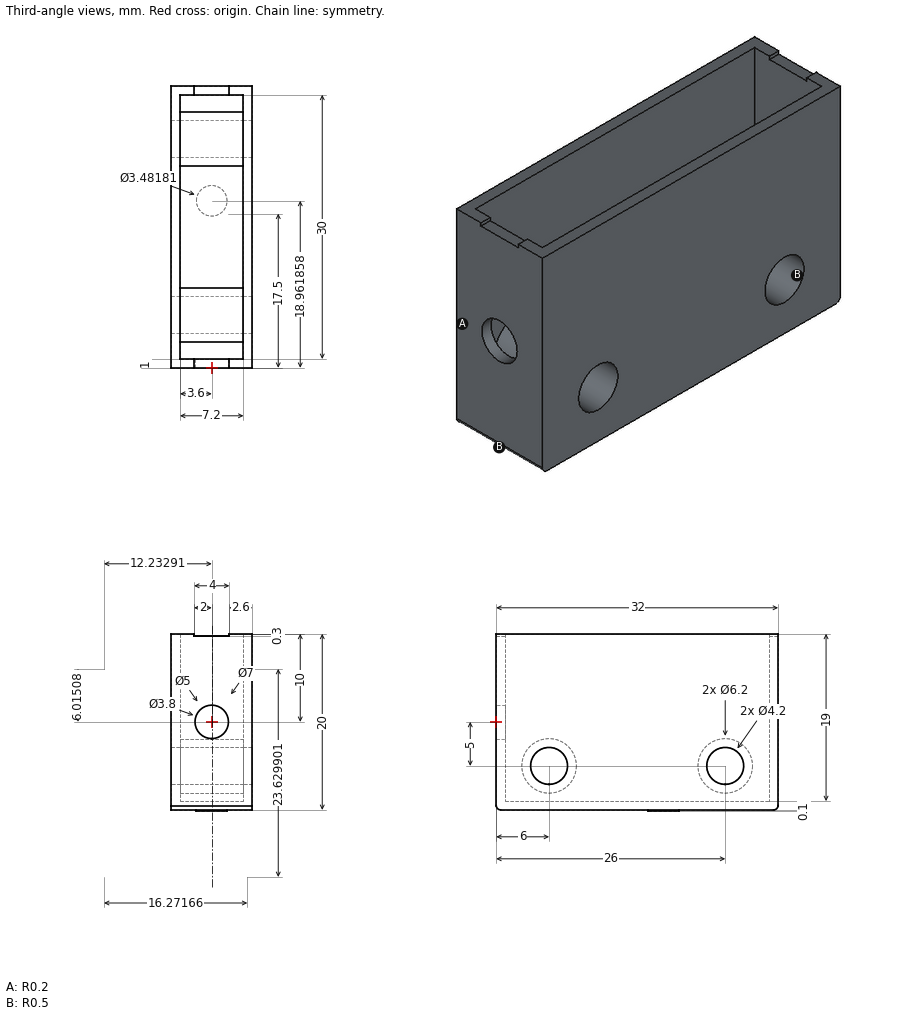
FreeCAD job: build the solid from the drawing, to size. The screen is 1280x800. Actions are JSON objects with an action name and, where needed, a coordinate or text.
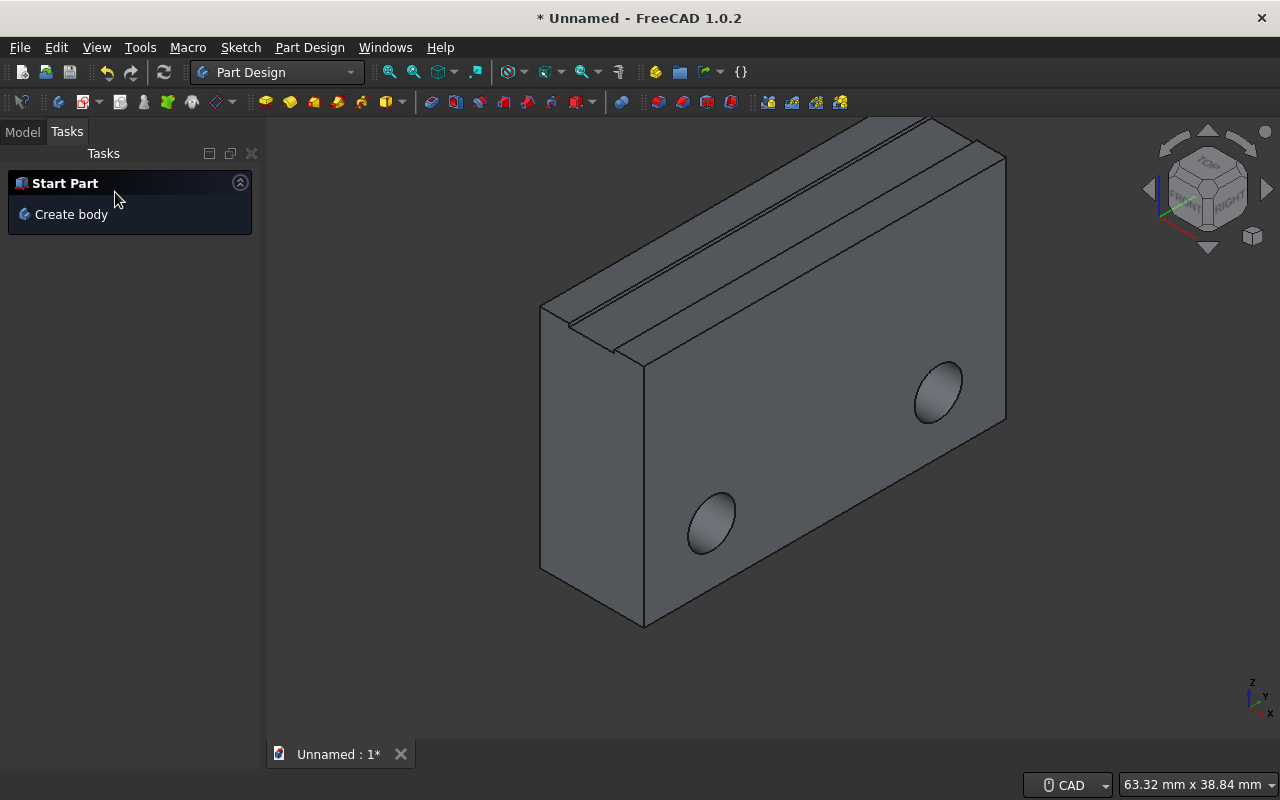
{"action": "left_click", "coordinate": [390, 72]}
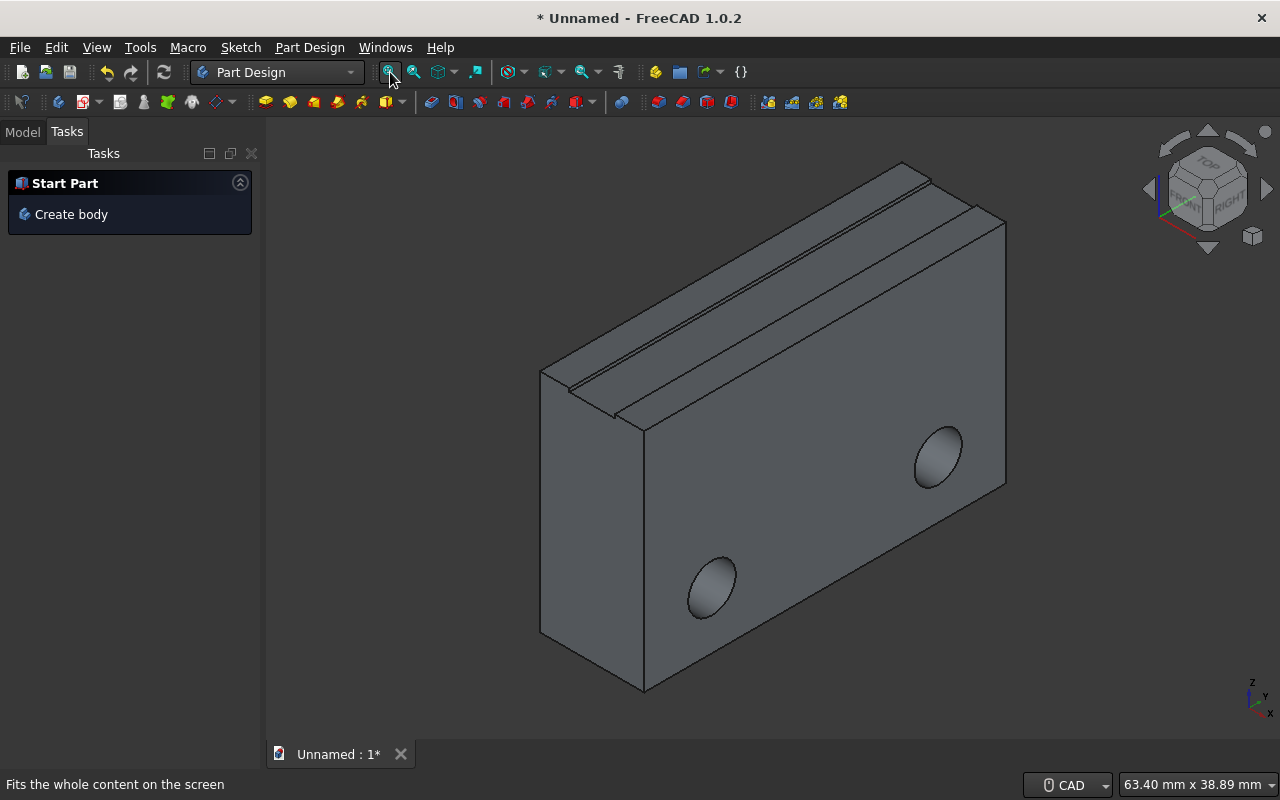
{"action": "left_click", "coordinate": [592, 494]}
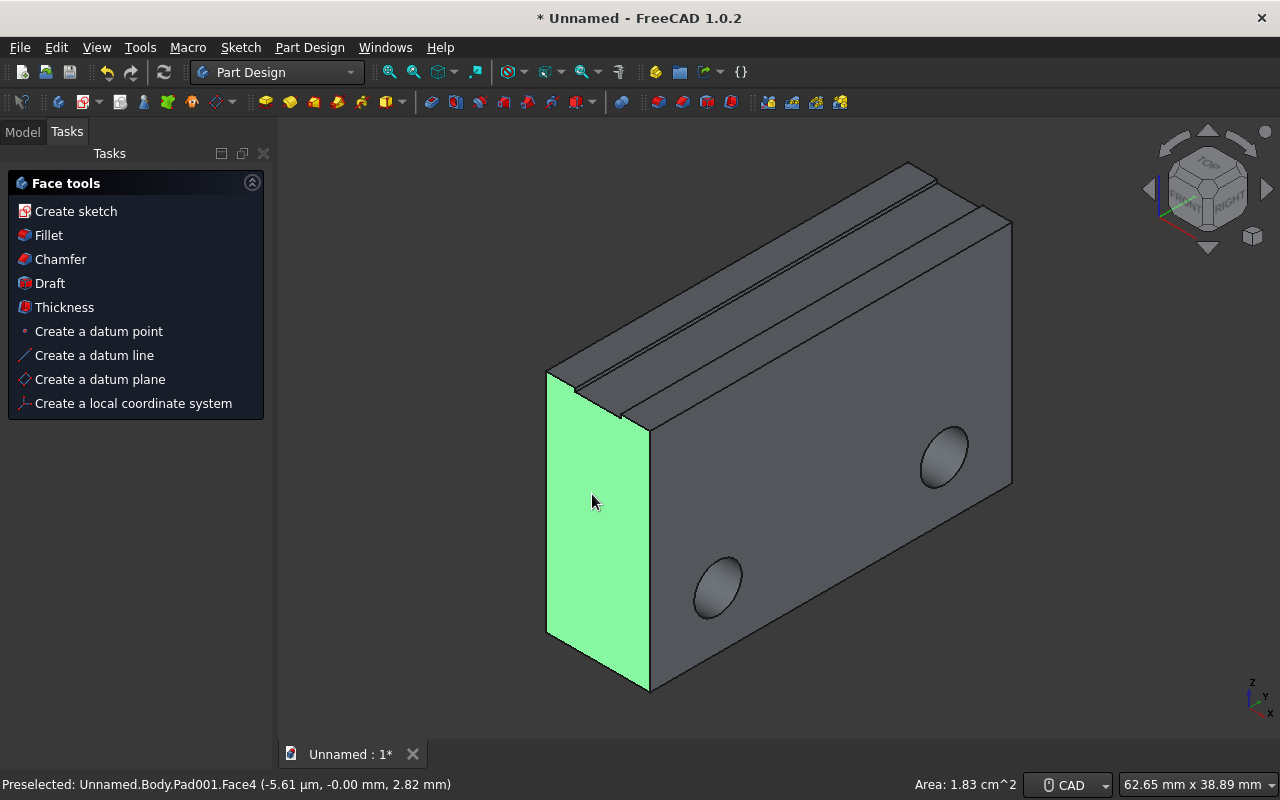
{"action": "left_click", "coordinate": [84, 102]}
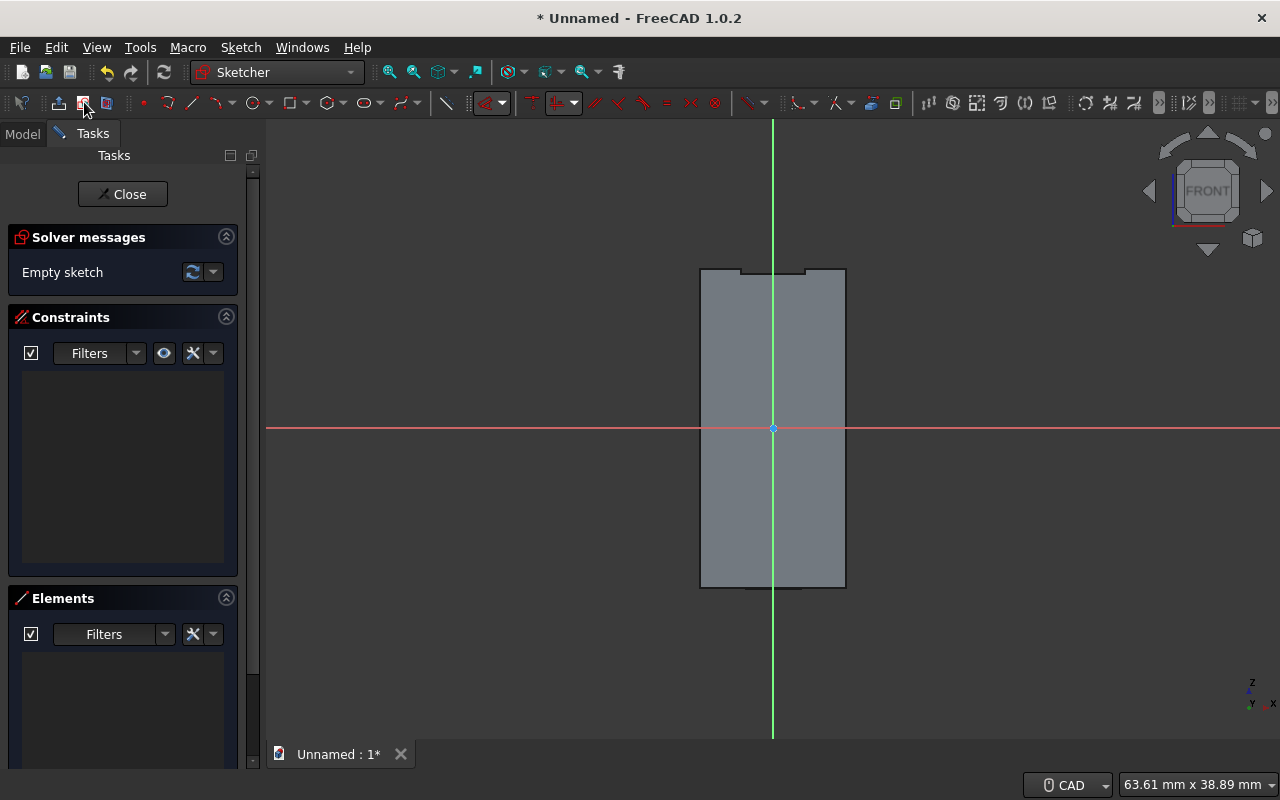
{"action": "scroll", "coordinate": [803, 428], "scroll_direction": "up", "scroll_amount": 6}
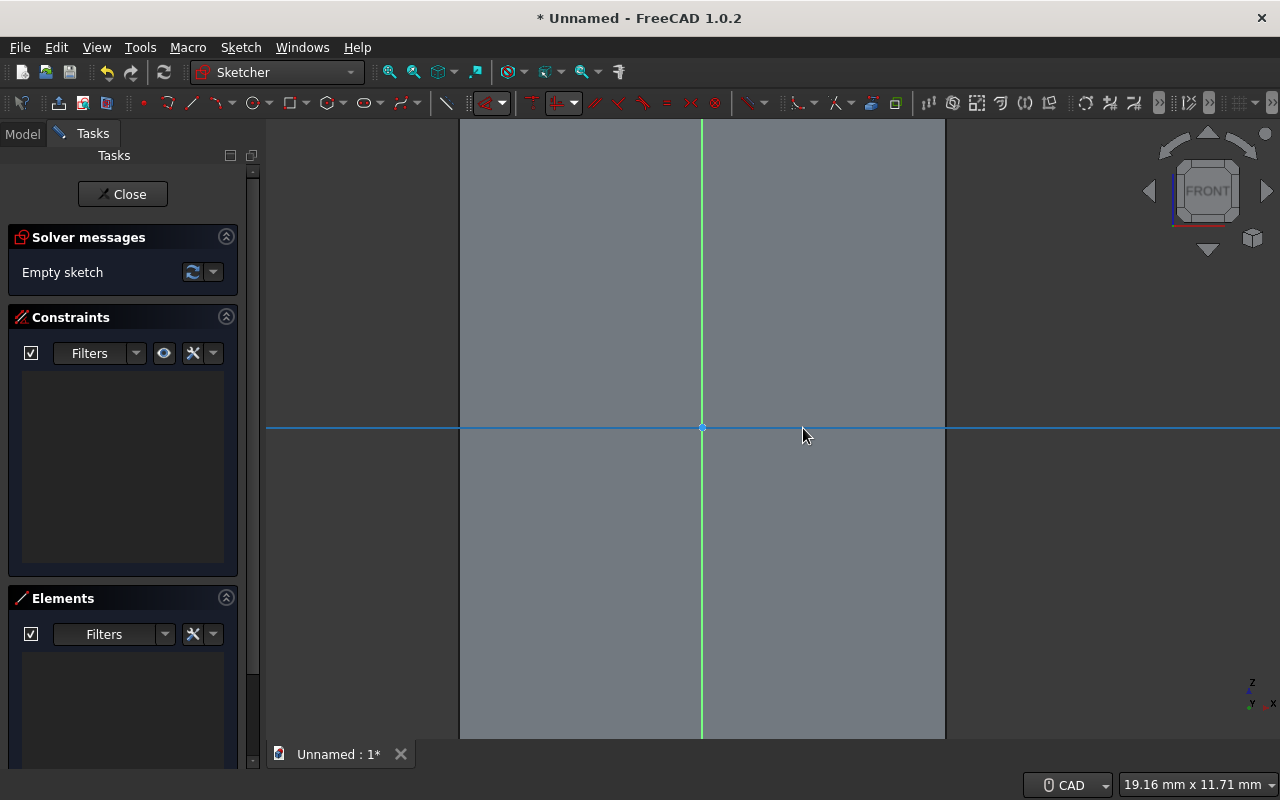
{"action": "left_click", "coordinate": [254, 104]}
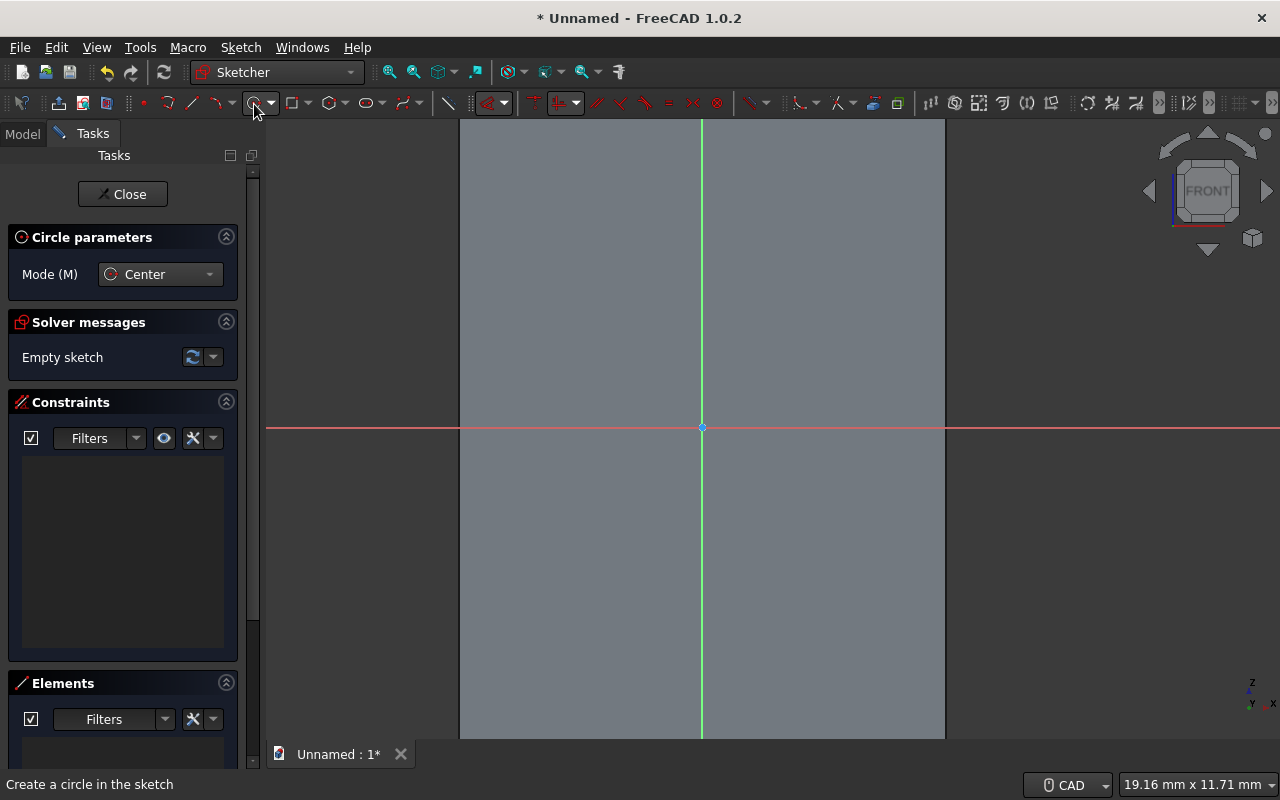
{"action": "left_click", "coordinate": [702, 428]}
{"action": "mouse_move", "coordinate": [833, 297]}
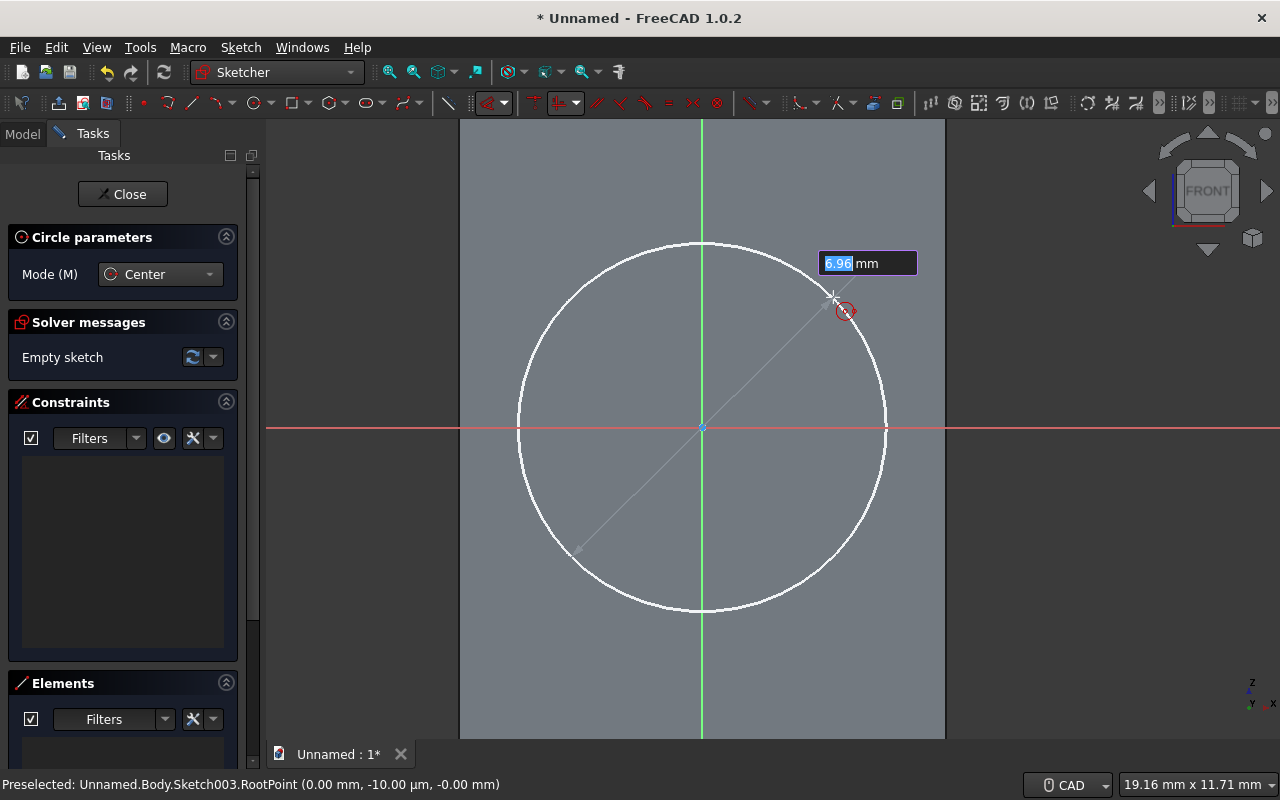
{"action": "type", "text": "7"}
{"action": "key", "text": "Return"}
{"action": "key", "text": "Escape"}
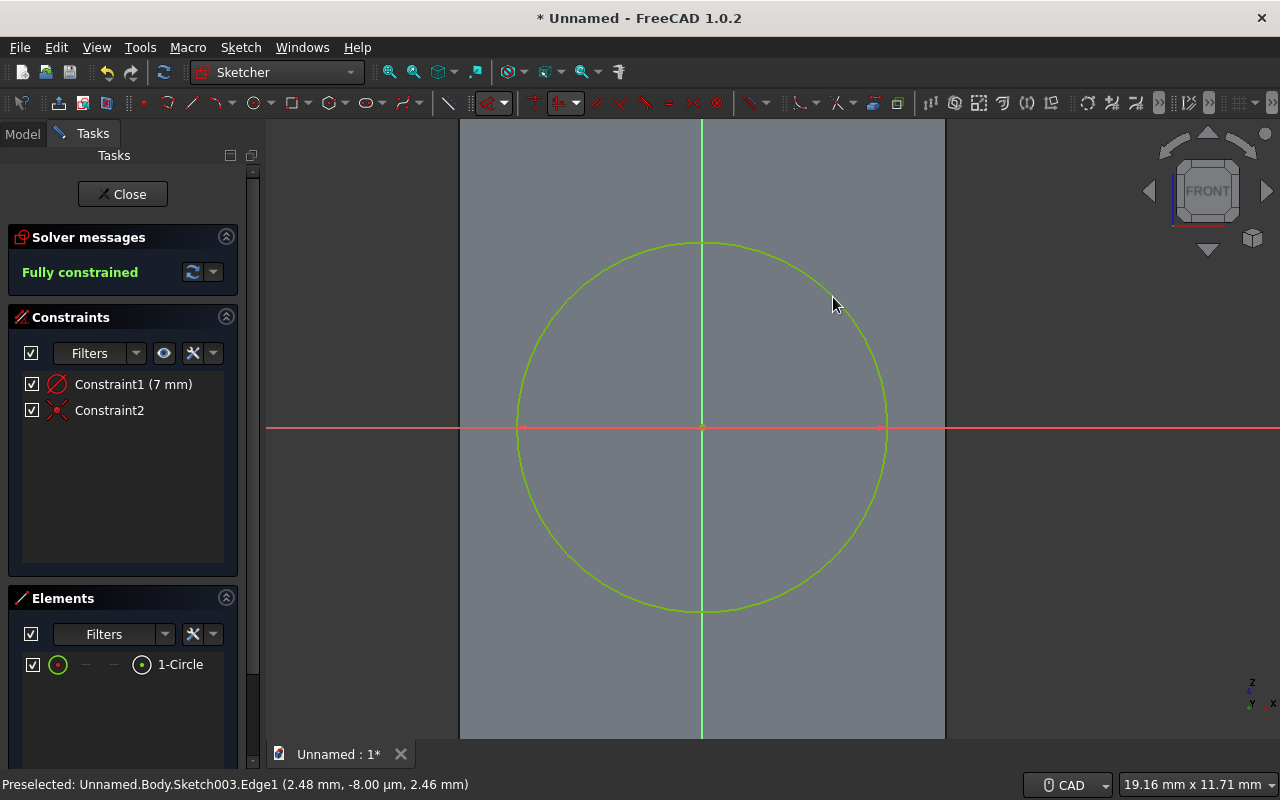
{"action": "left_click", "coordinate": [123, 194]}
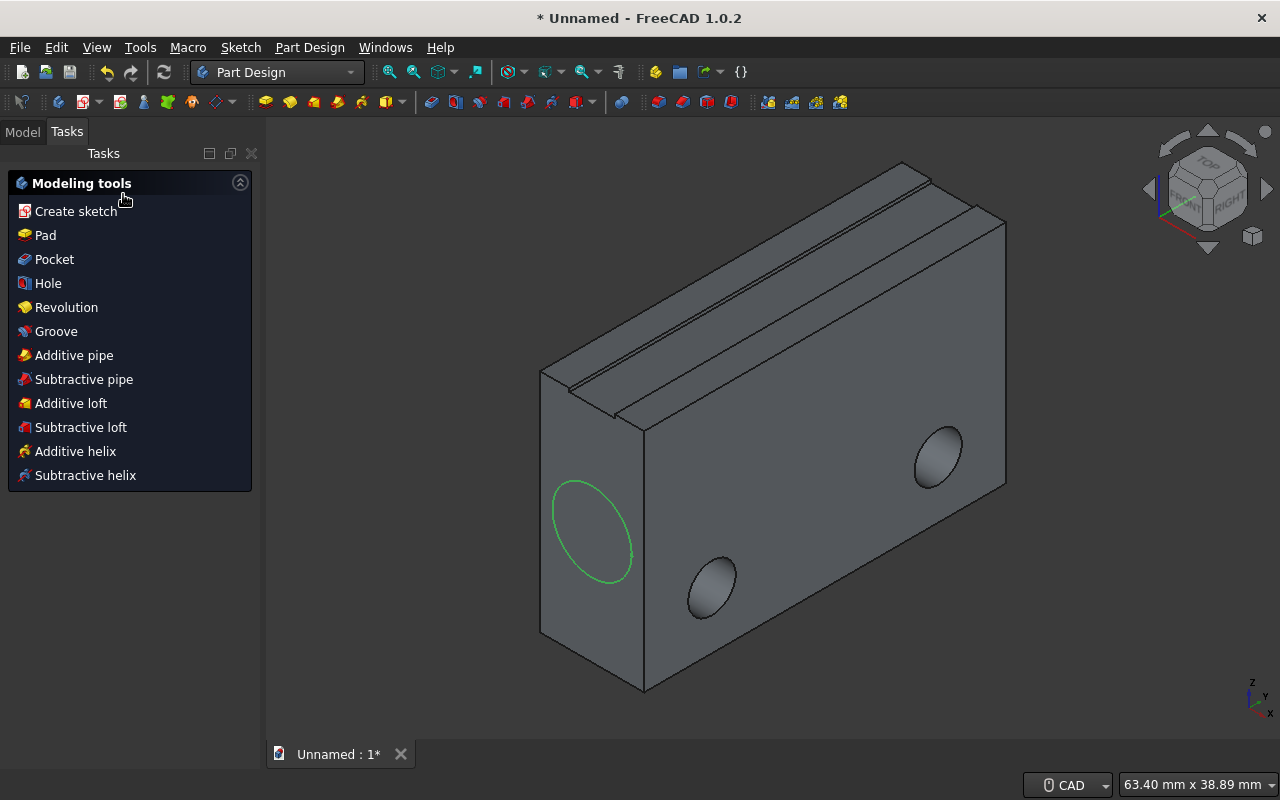
{"action": "left_click", "coordinate": [266, 102]}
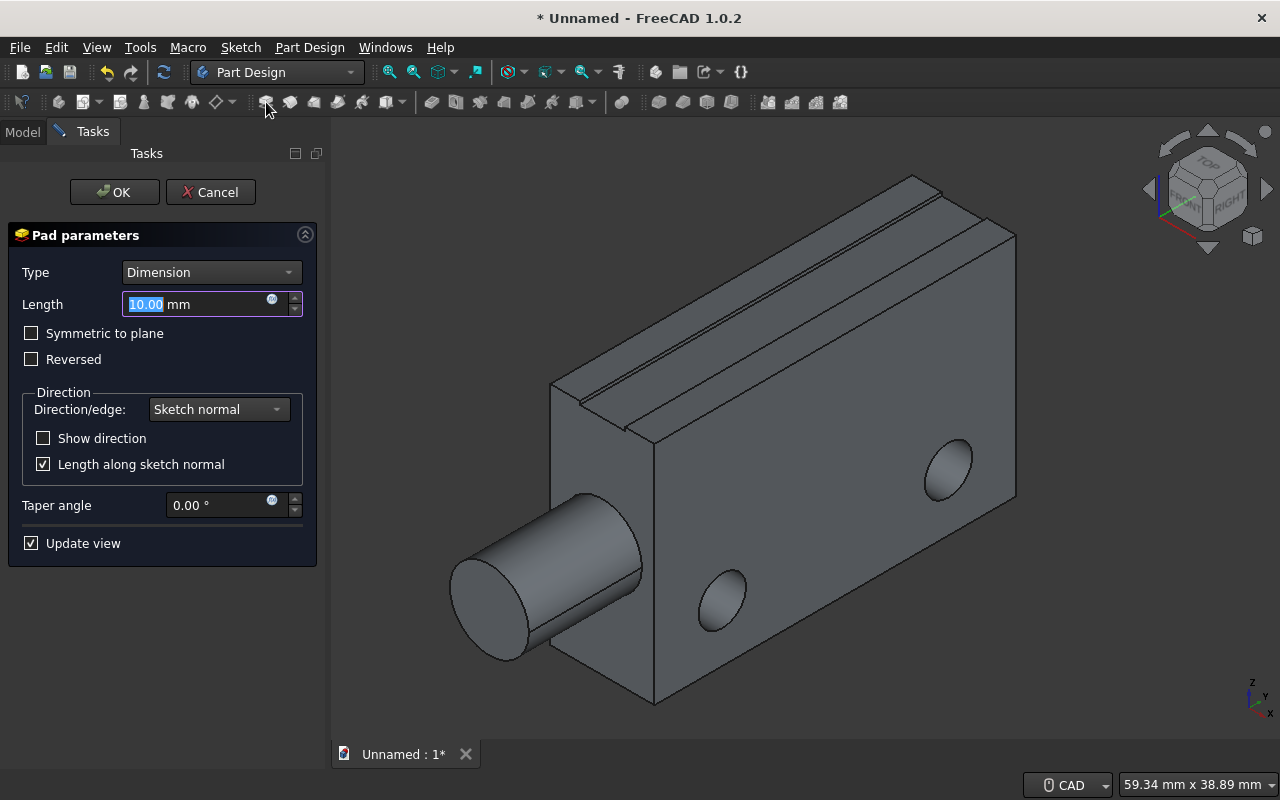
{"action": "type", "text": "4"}
{"action": "key", "text": "Tab"}